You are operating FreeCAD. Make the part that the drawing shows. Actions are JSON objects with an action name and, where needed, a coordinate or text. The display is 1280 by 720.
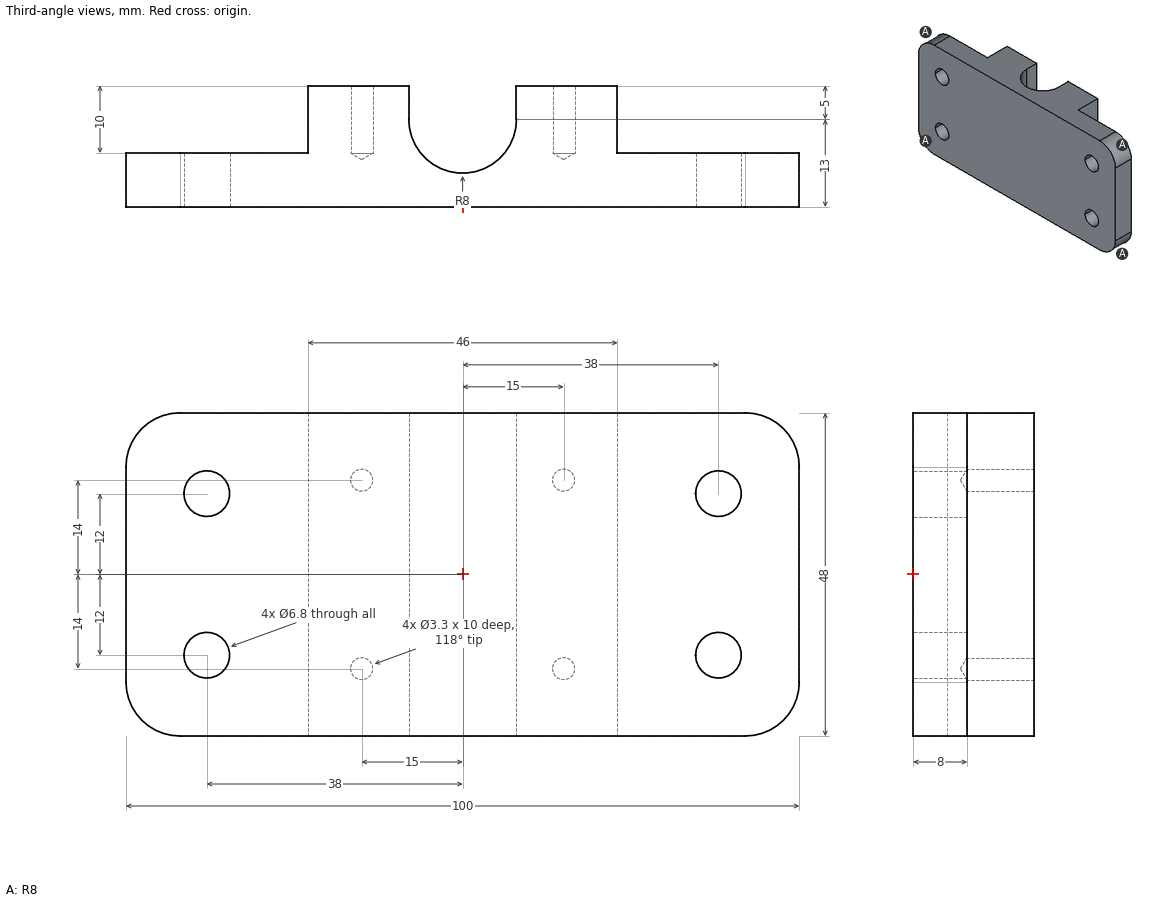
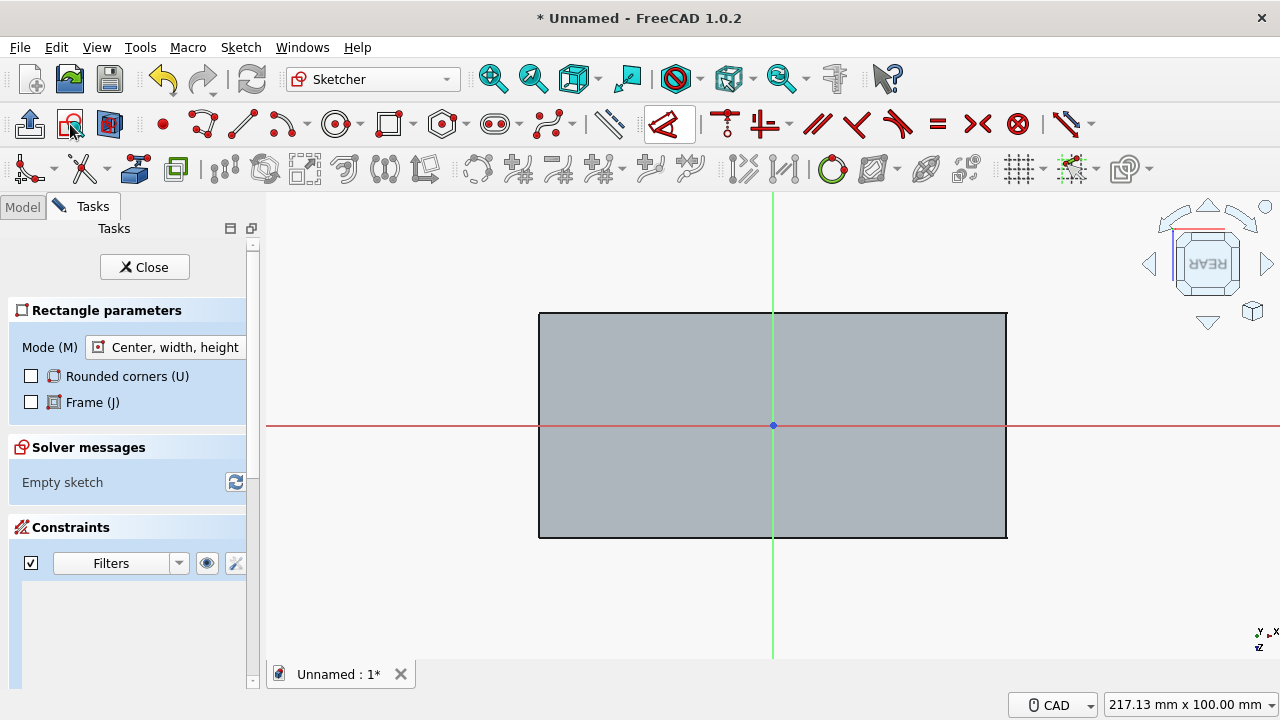
{"action": "left_click", "coordinate": [773, 426]}
{"action": "left_click", "coordinate": [880, 313]}
{"action": "key", "text": "Escape"}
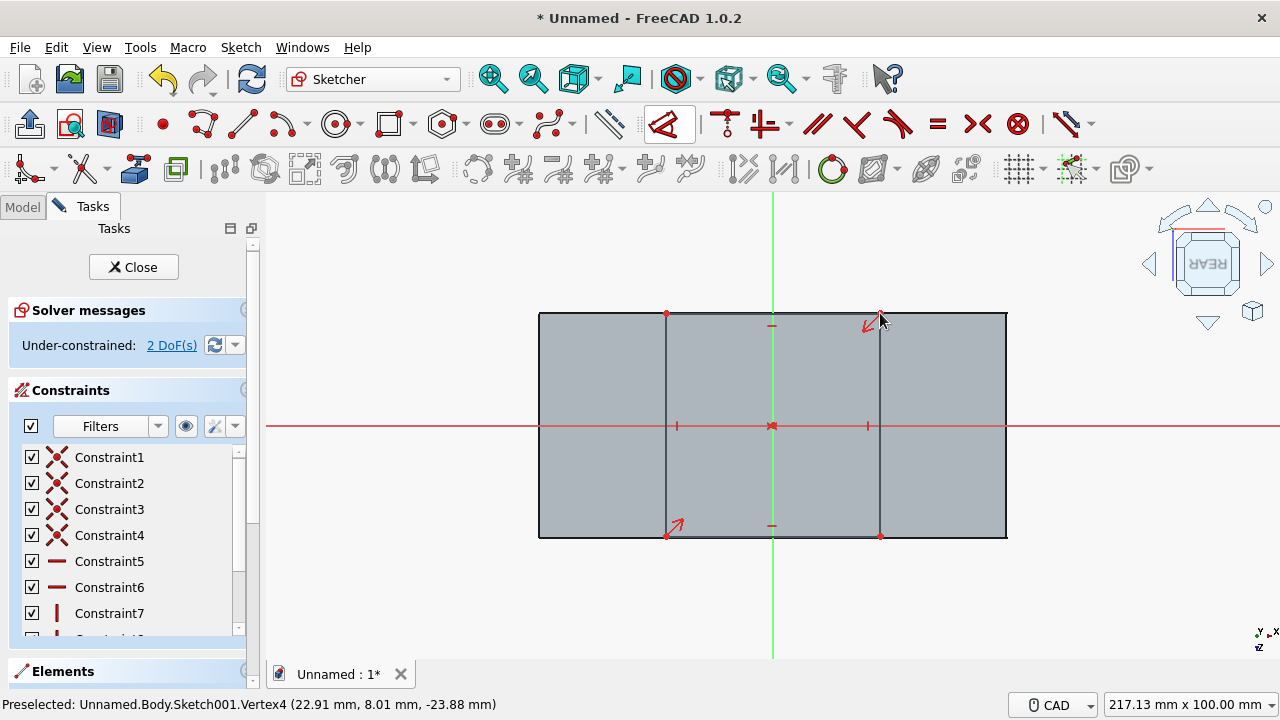
{"action": "left_click", "coordinate": [730, 537]}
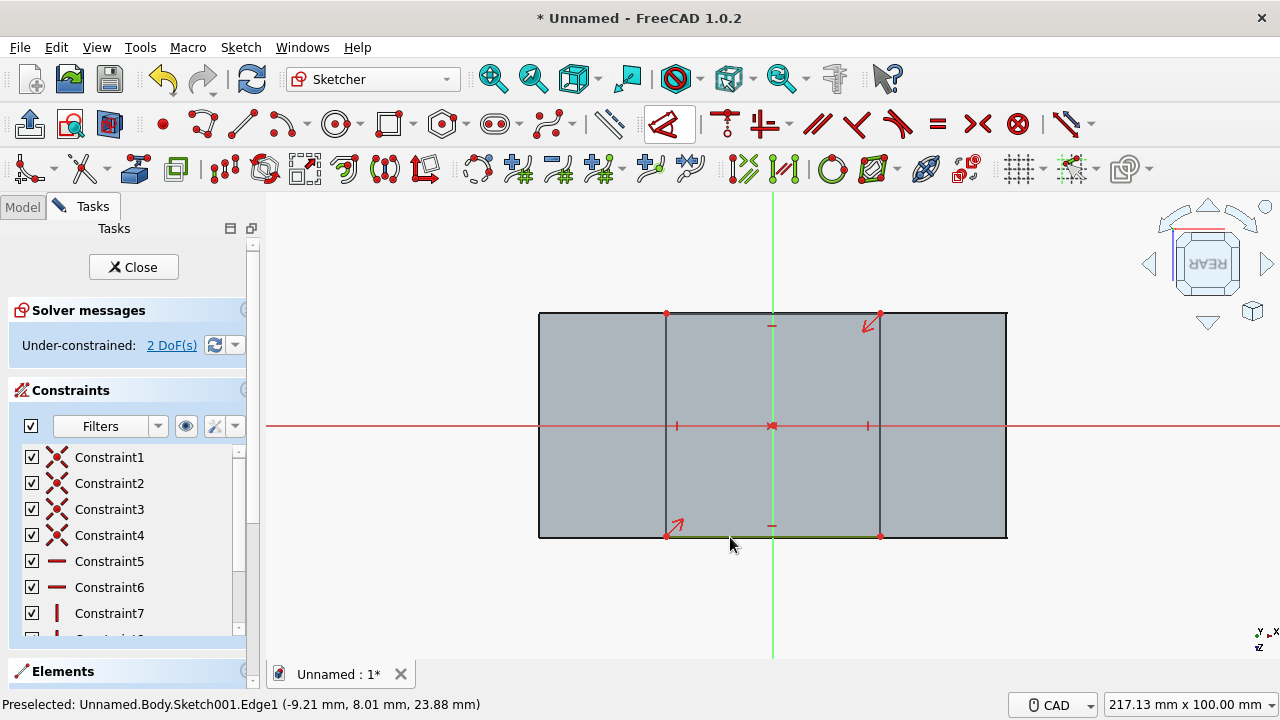
{"action": "left_click", "coordinate": [690, 124]}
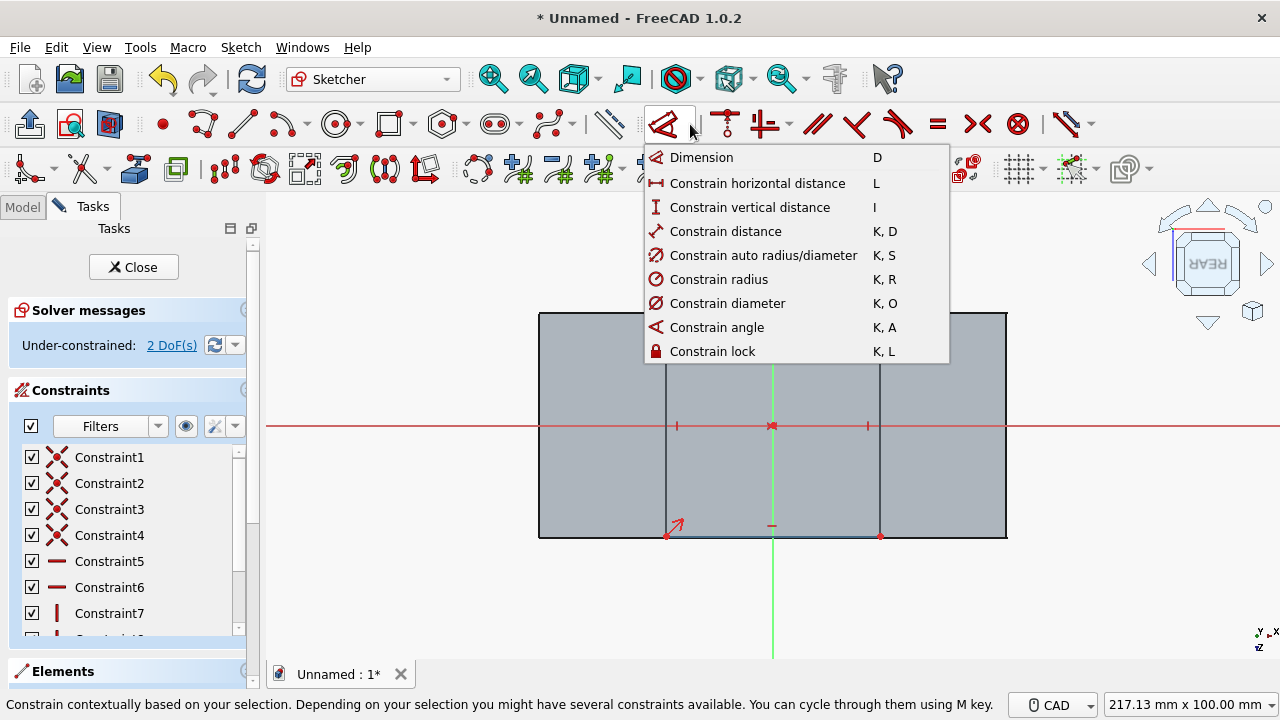
{"action": "left_click", "coordinate": [797, 183]}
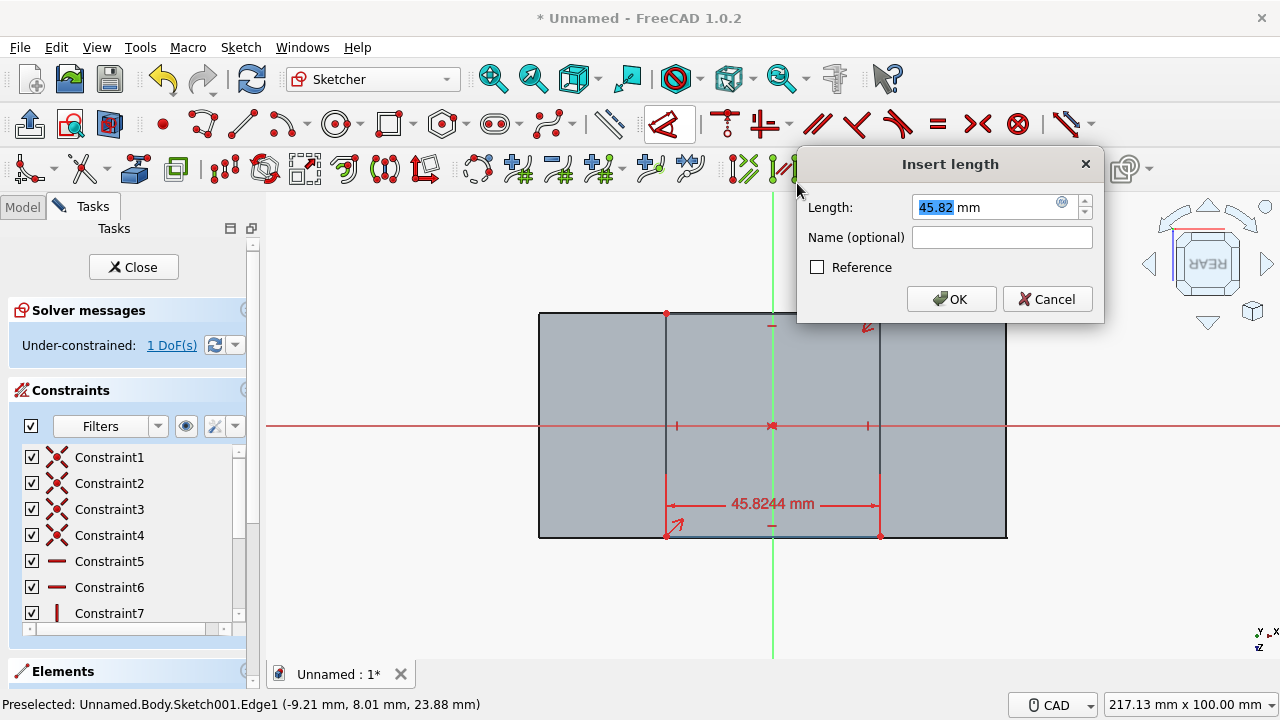
{"action": "type", "text": "46"}
{"action": "key", "text": "Return"}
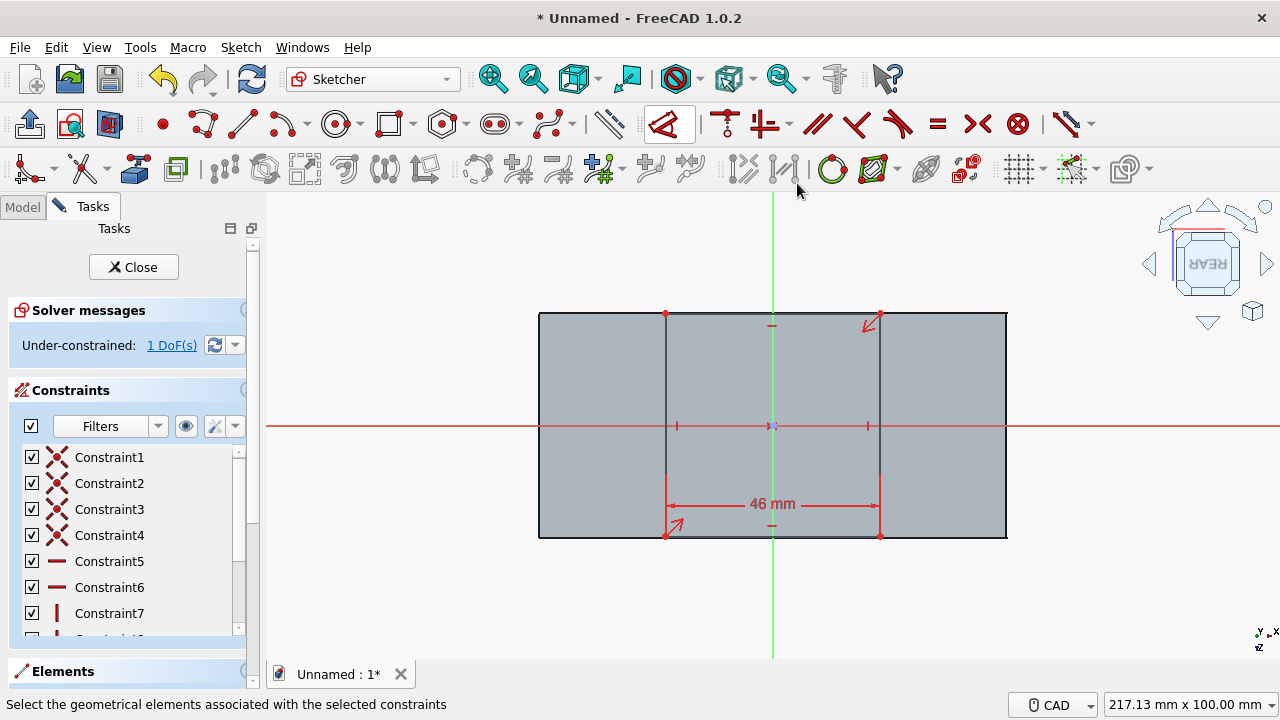
{"action": "left_click", "coordinate": [880, 470]}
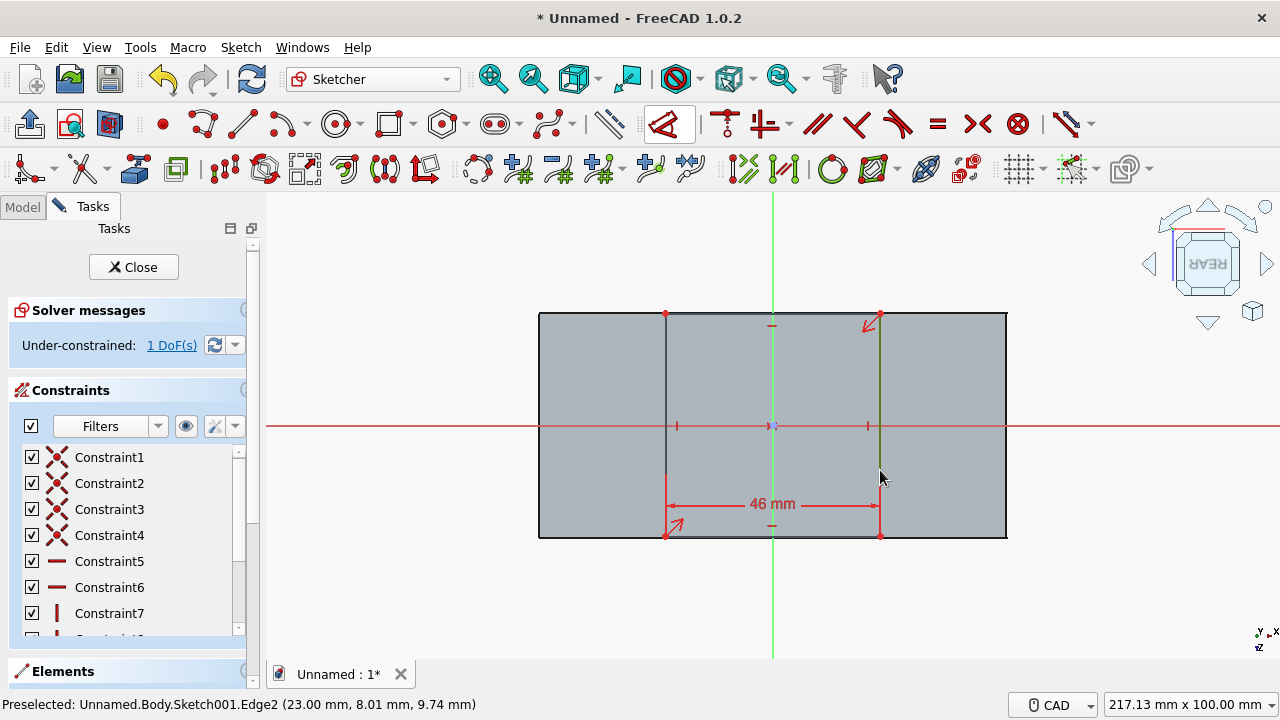
{"action": "key", "text": "i"}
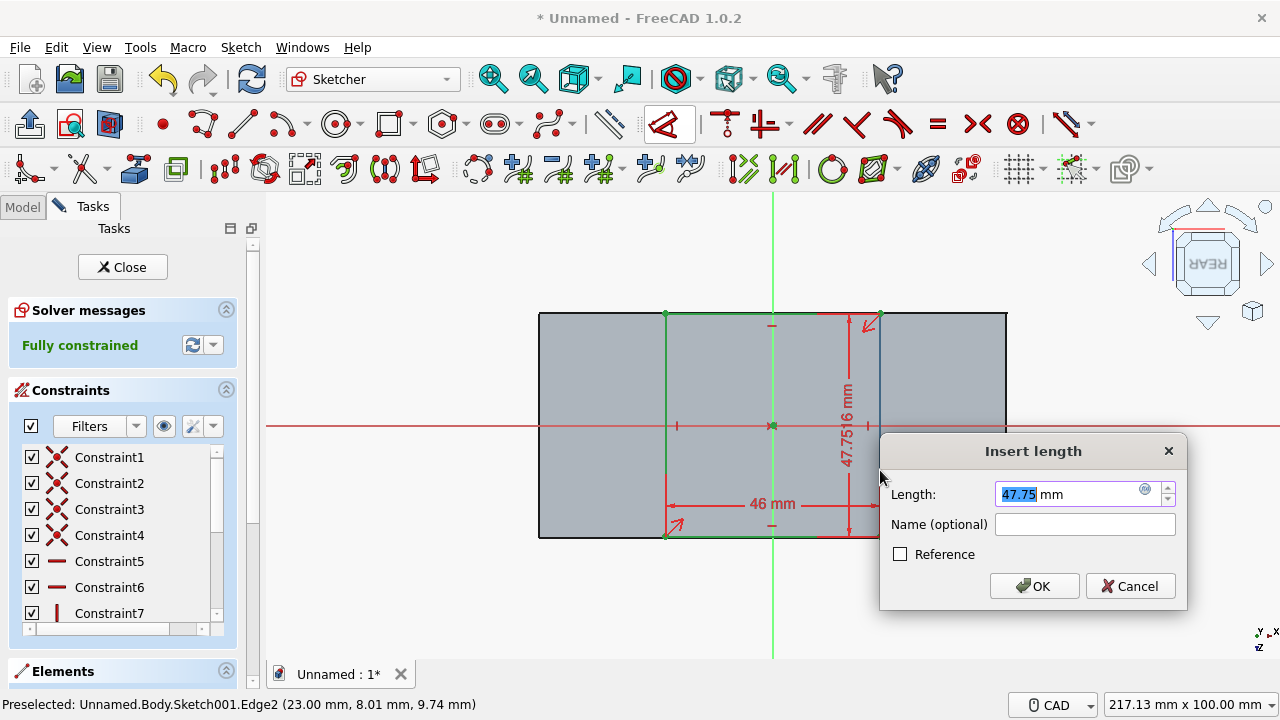
{"action": "type", "text": "48"}
{"action": "key", "text": "Return"}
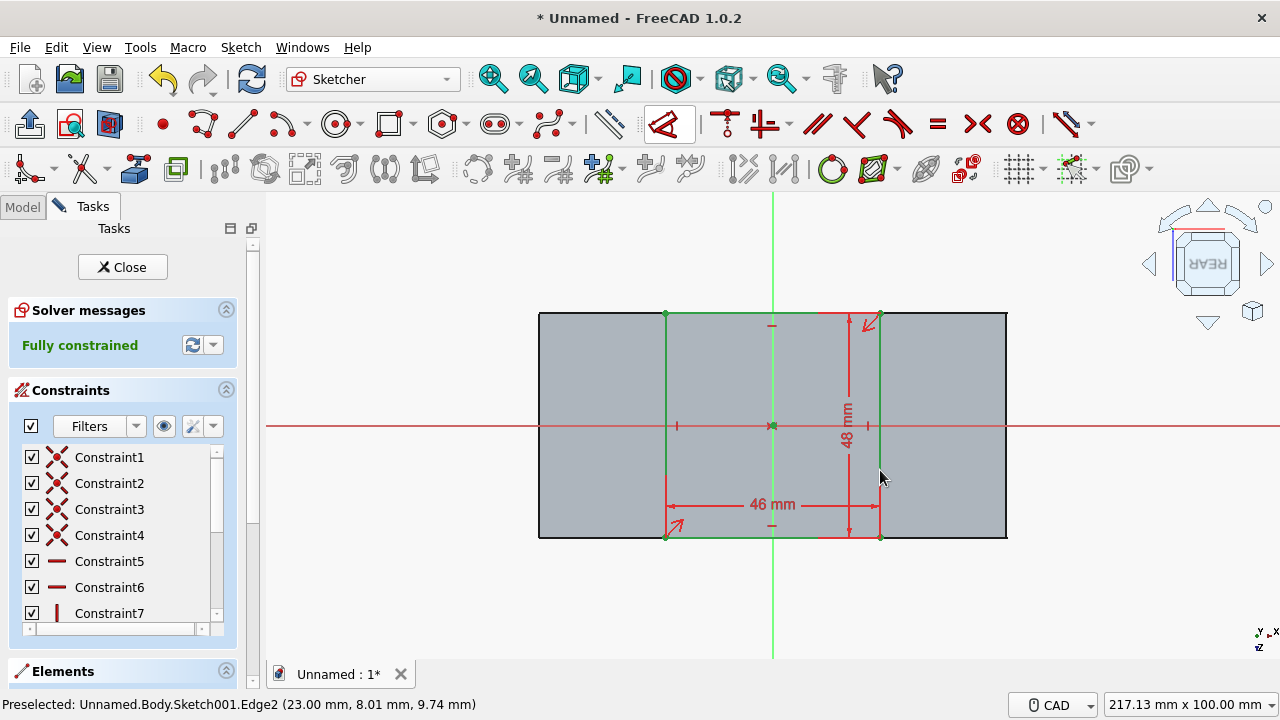
{"action": "left_click", "coordinate": [123, 267]}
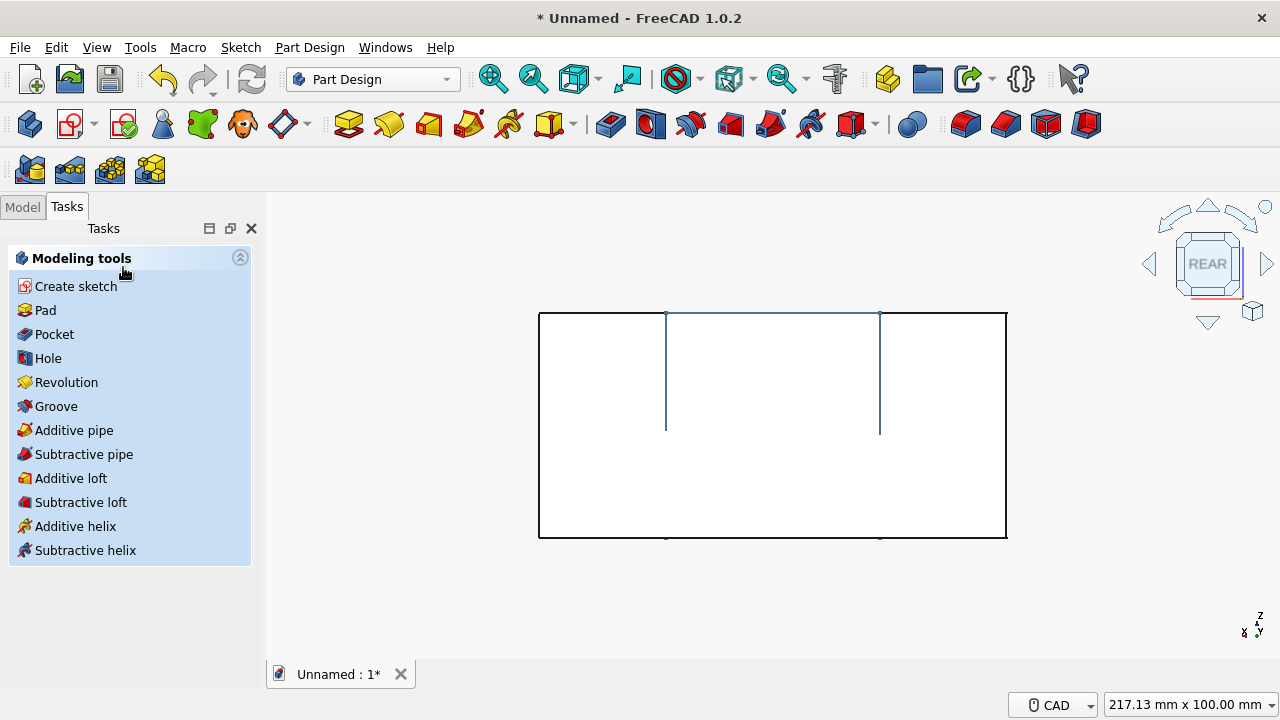
{"action": "left_click", "coordinate": [350, 124]}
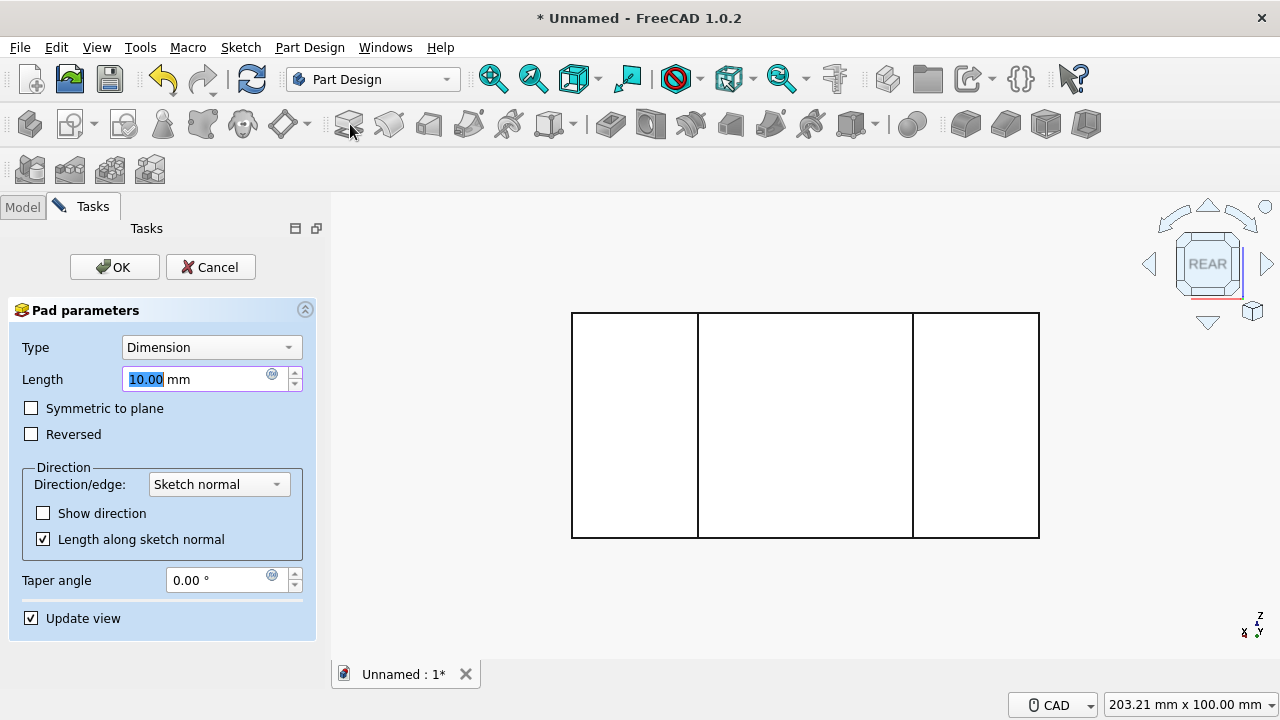
{"action": "type", "text": "10"}
{"action": "key", "text": "Tab"}